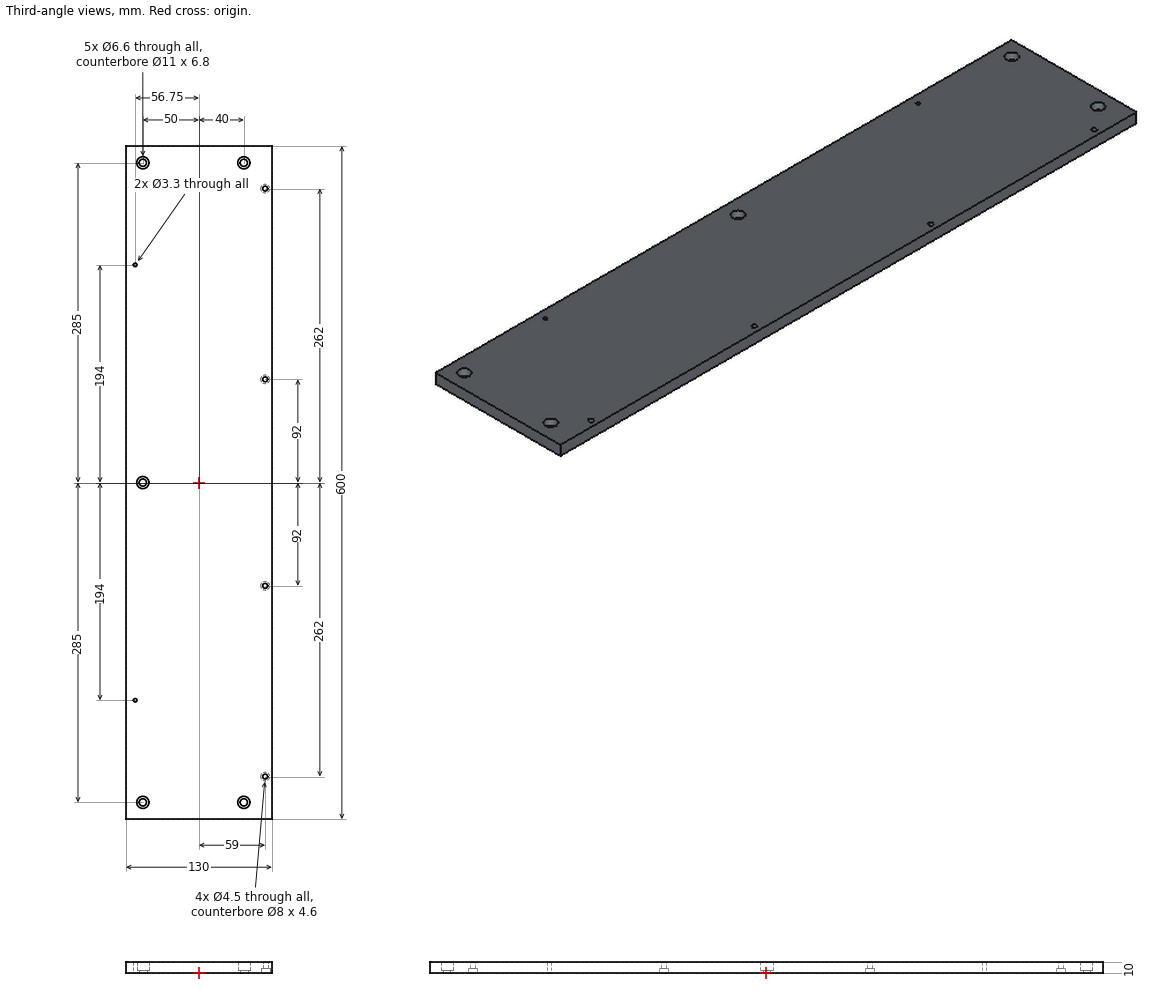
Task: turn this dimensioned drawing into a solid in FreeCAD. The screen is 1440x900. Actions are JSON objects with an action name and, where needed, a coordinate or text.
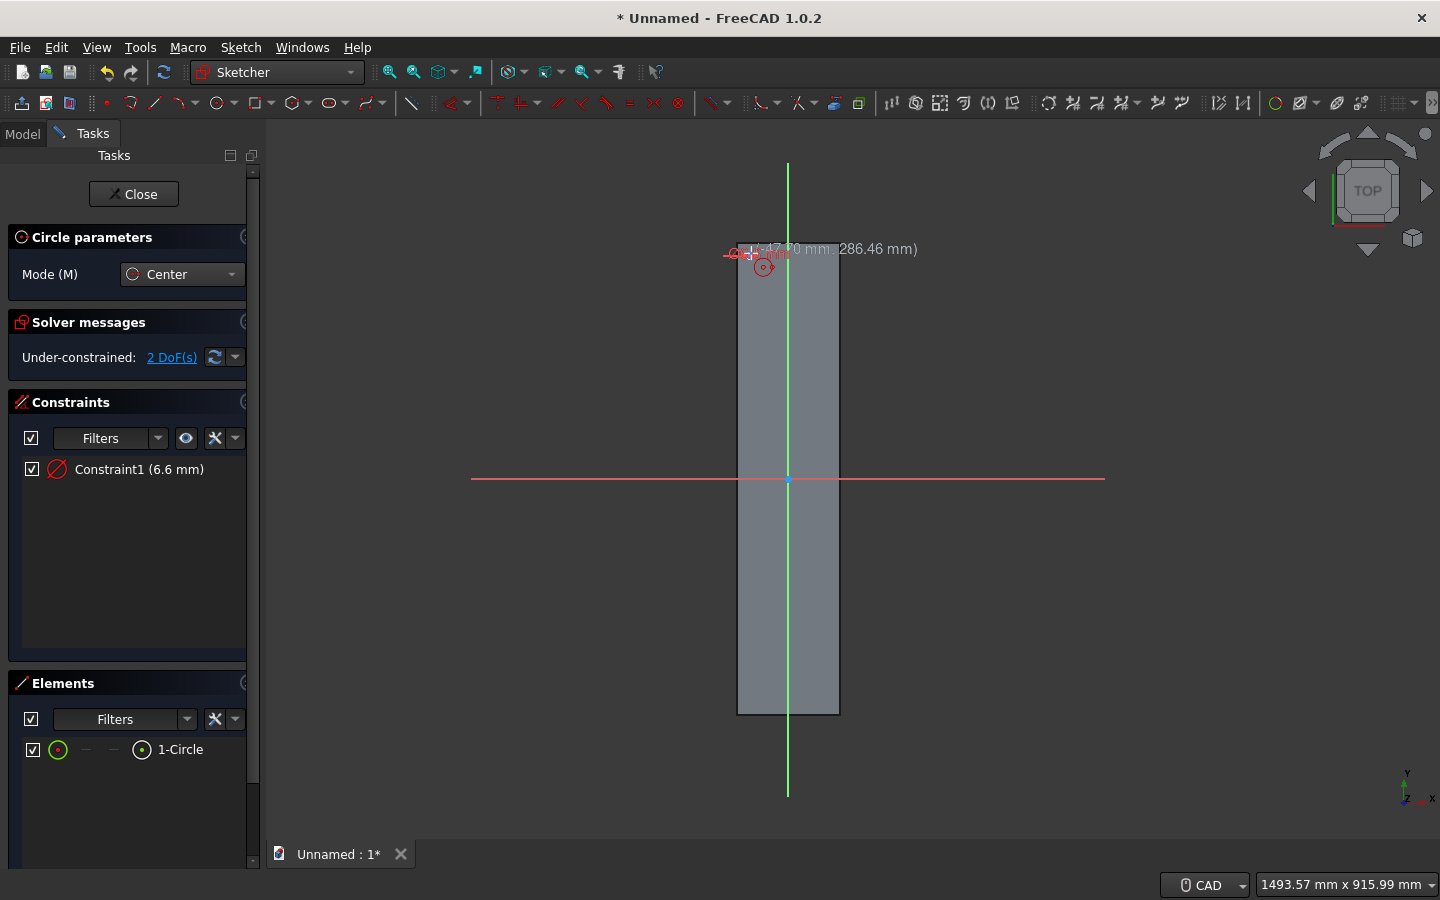
{"action": "scroll", "coordinate": [749, 479], "scroll_direction": "up", "scroll_amount": 11}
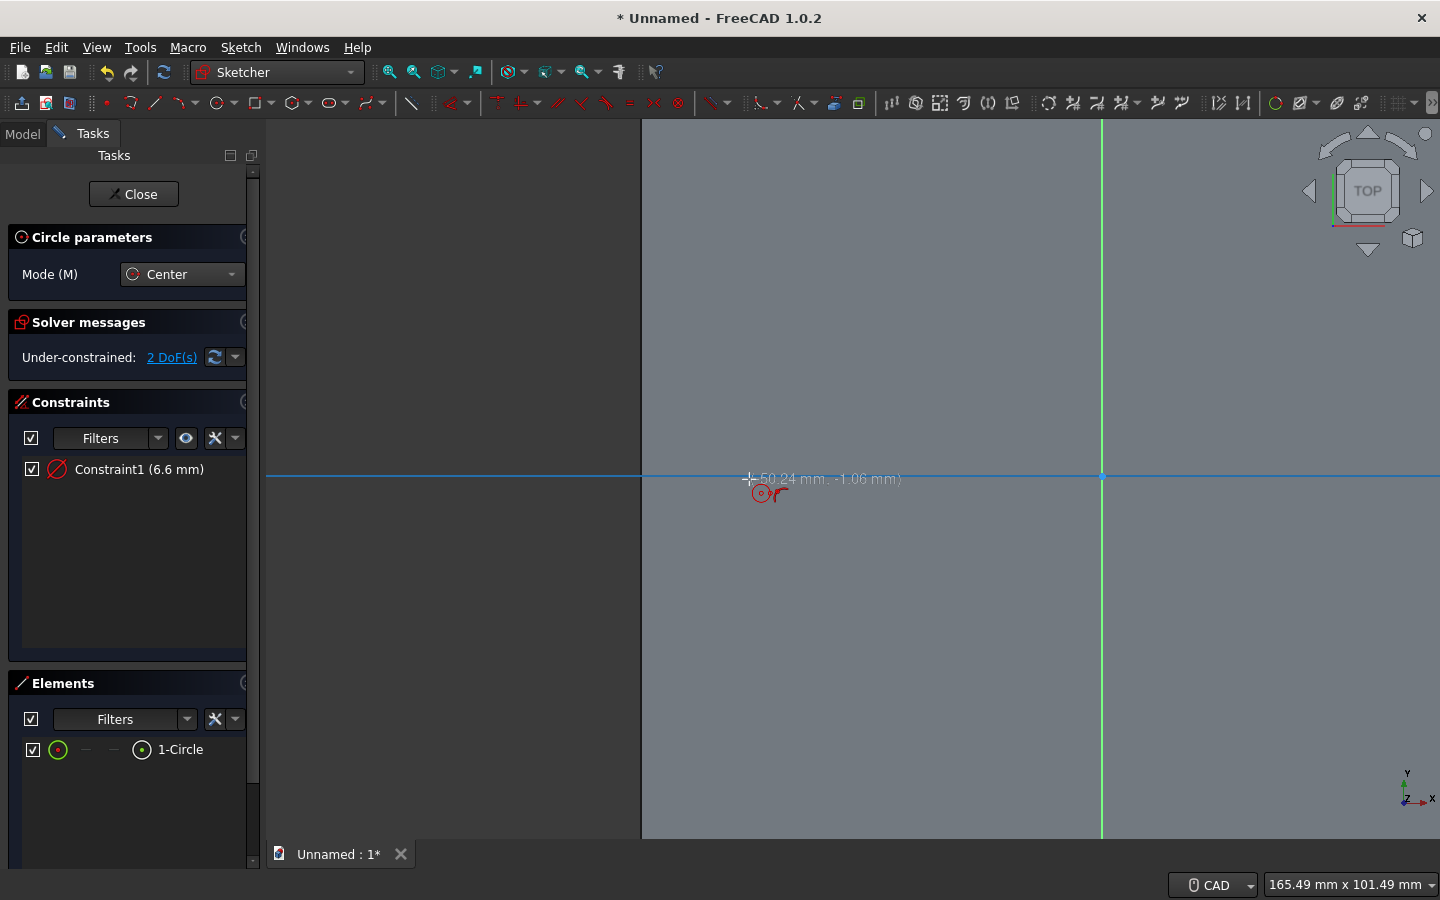
{"action": "scroll", "coordinate": [749, 479], "scroll_direction": "down", "scroll_amount": 11}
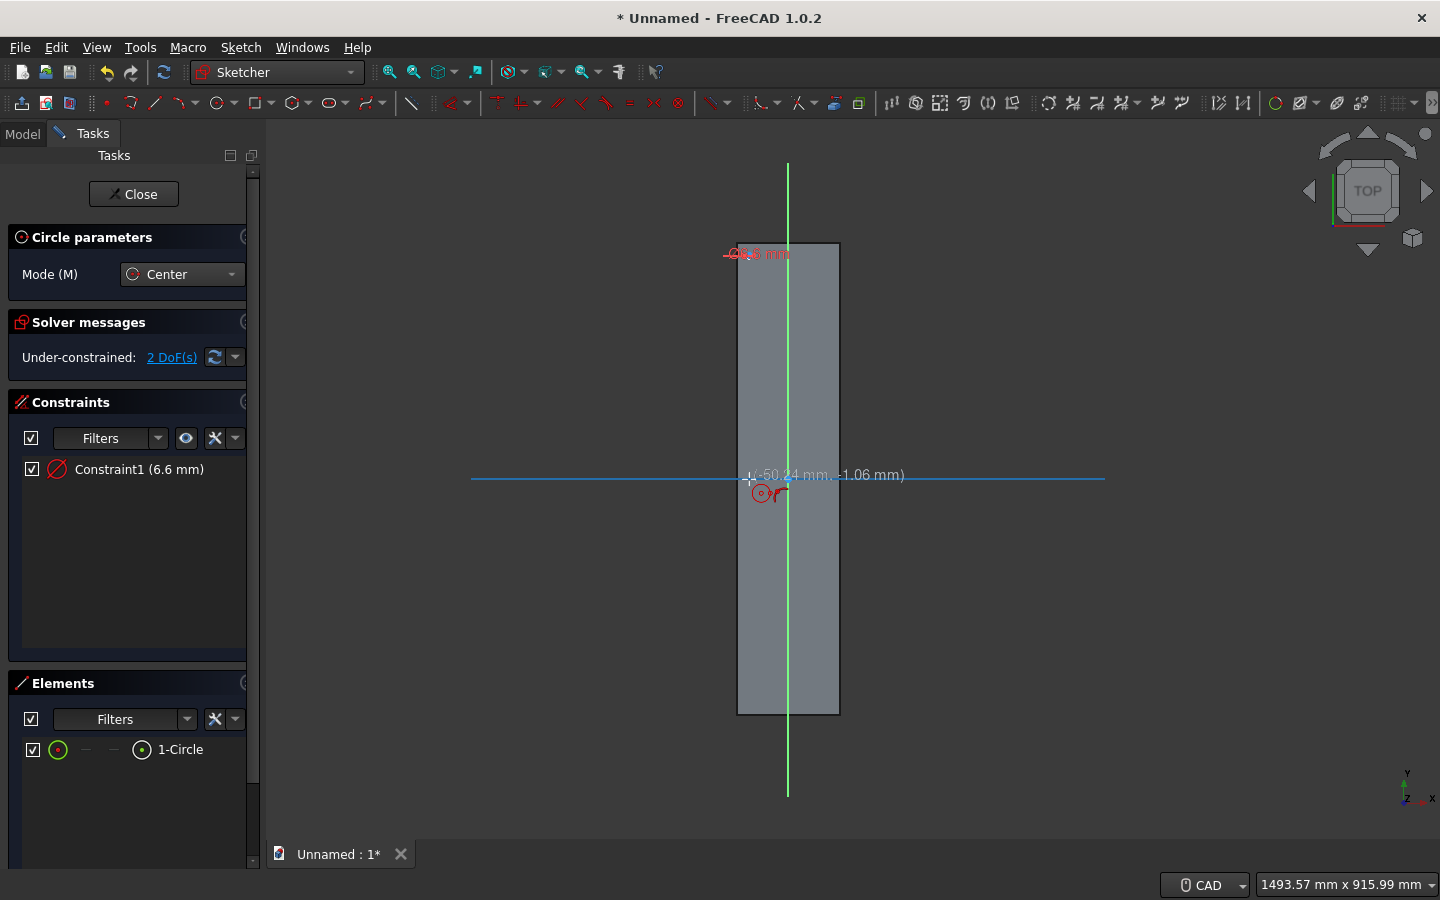
{"action": "left_click", "coordinate": [749, 479]}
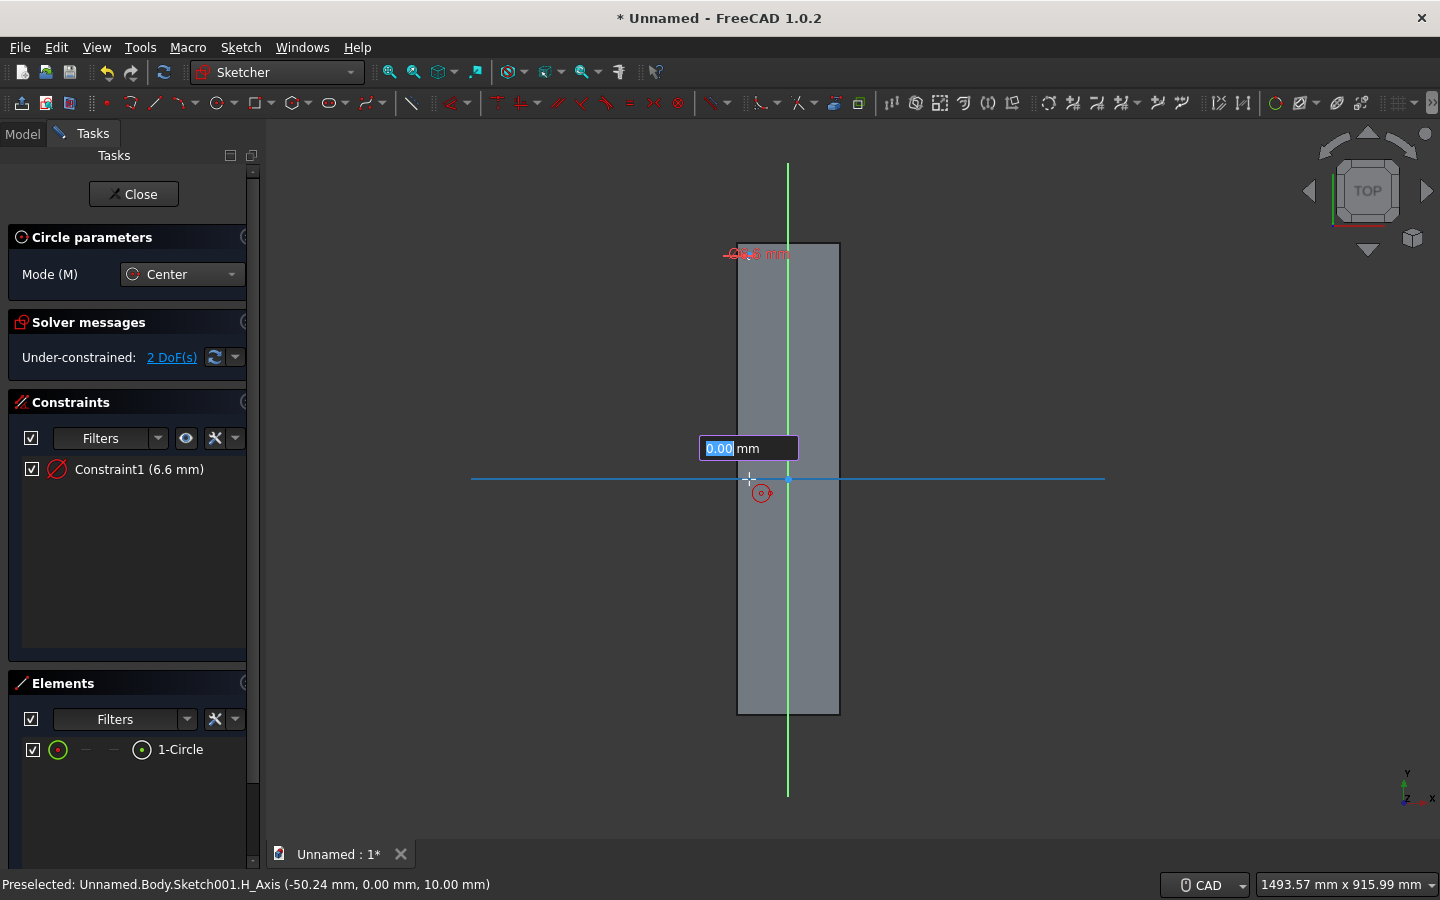
{"action": "scroll", "coordinate": [748, 482], "scroll_direction": "up", "scroll_amount": 10}
{"action": "mouse_move", "coordinate": [748, 476]}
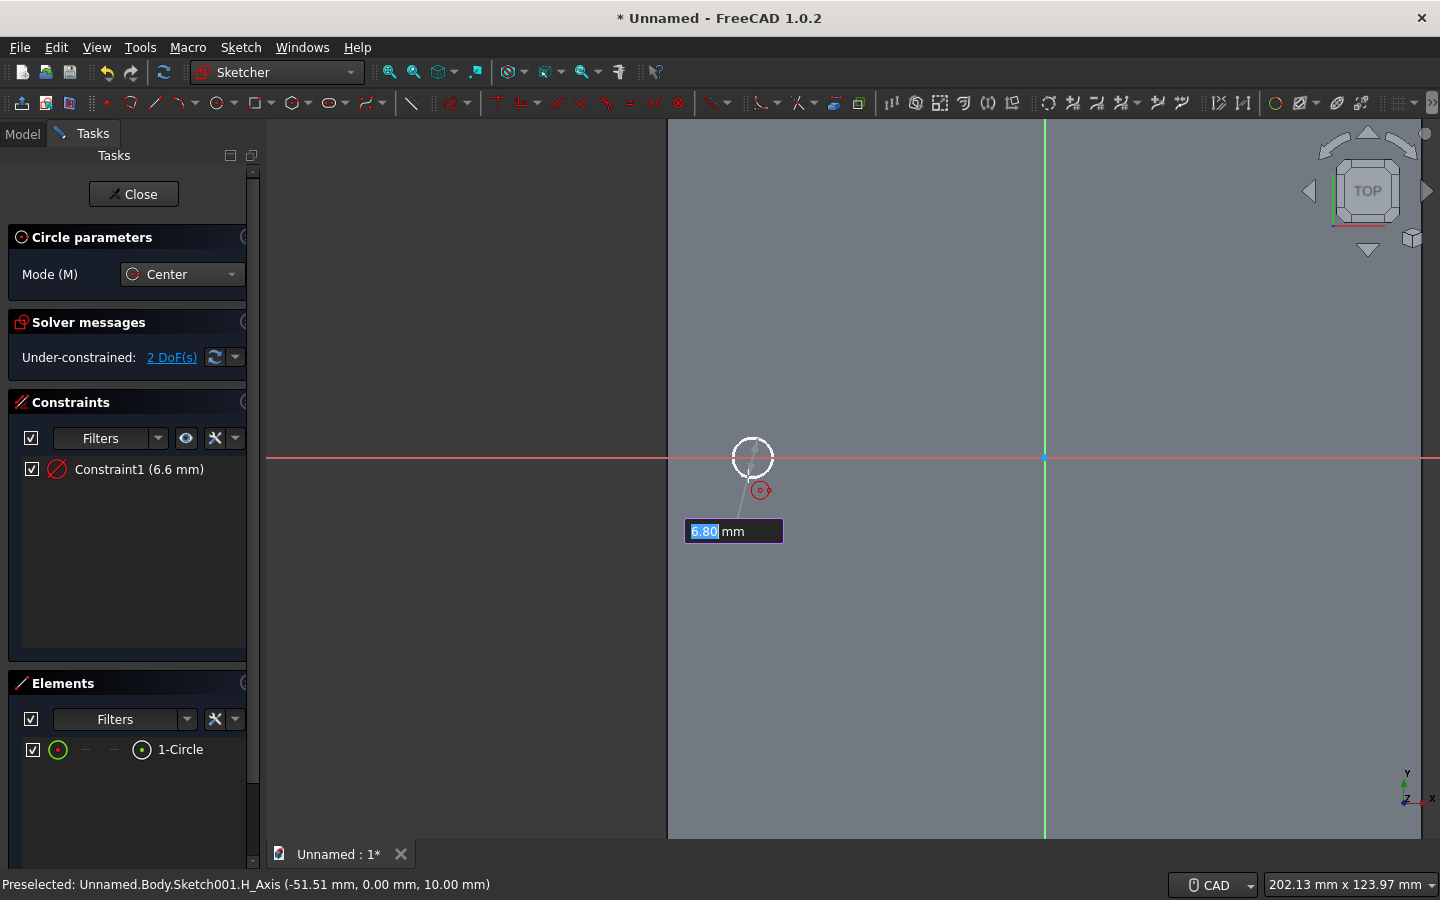
{"action": "type", "text": "6.6"}
{"action": "key", "text": "Return"}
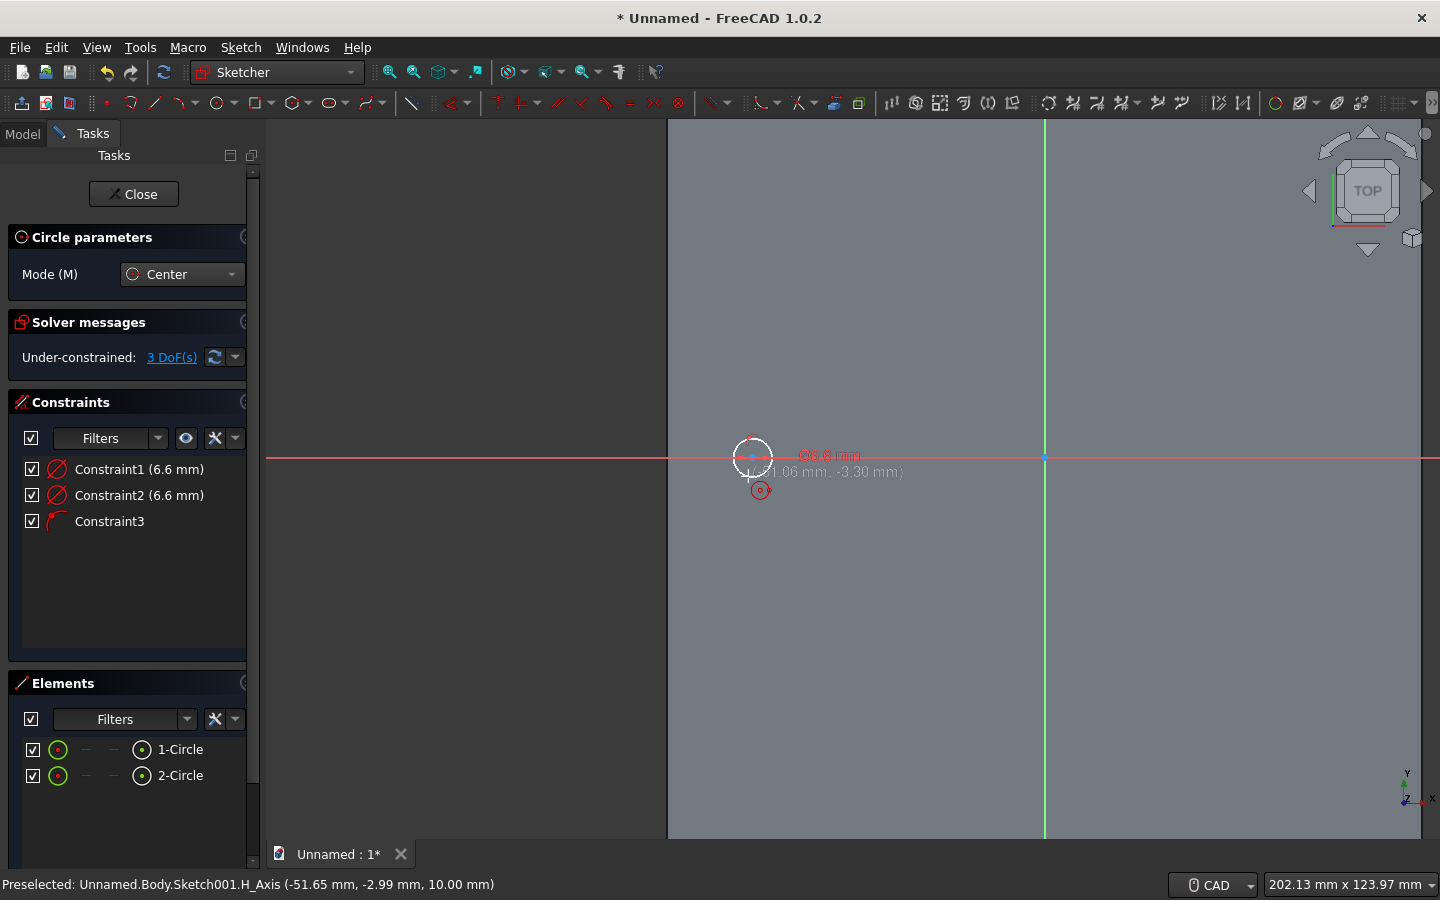
{"action": "scroll", "coordinate": [748, 482], "scroll_direction": "down", "scroll_amount": 10}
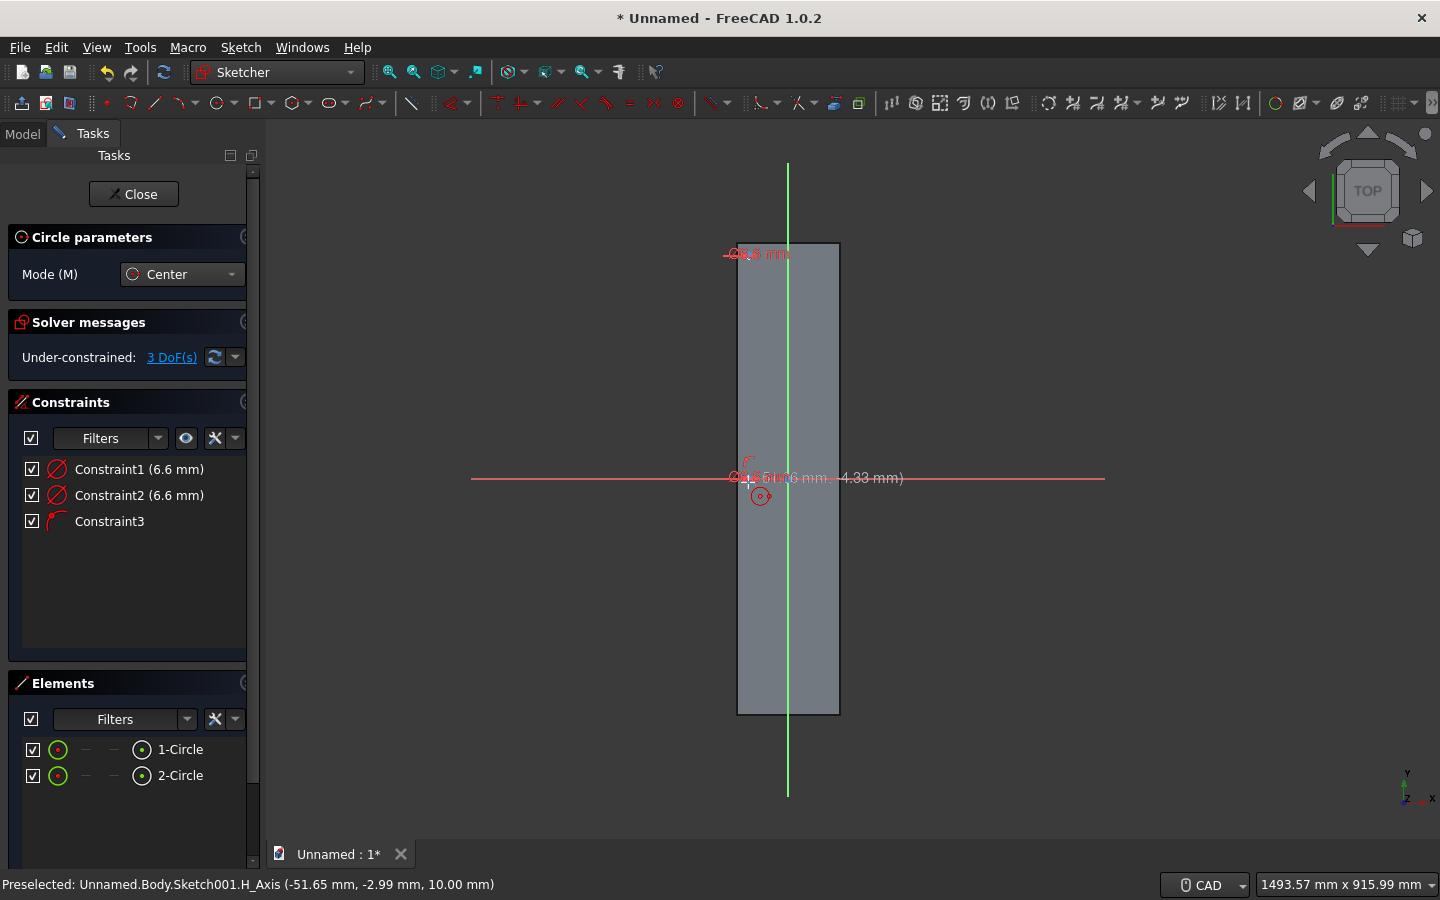
{"action": "scroll", "coordinate": [749, 703], "scroll_direction": "up", "scroll_amount": 11}